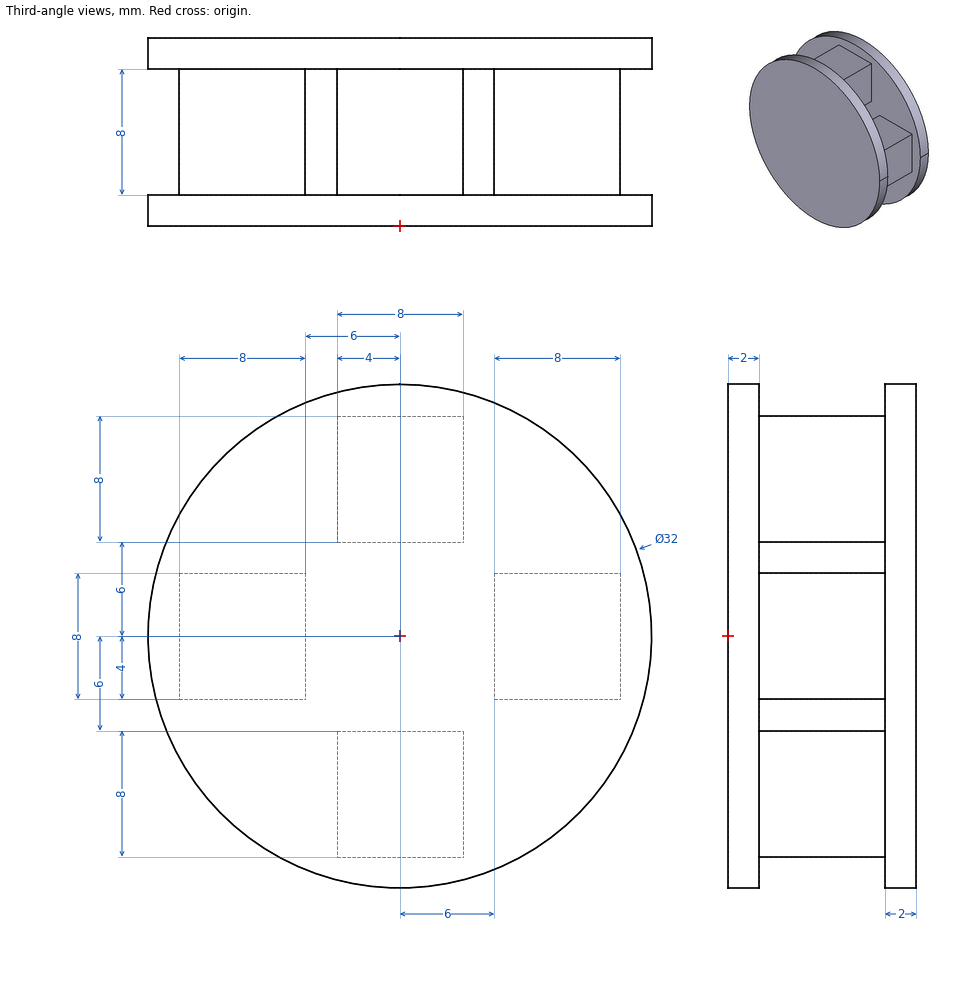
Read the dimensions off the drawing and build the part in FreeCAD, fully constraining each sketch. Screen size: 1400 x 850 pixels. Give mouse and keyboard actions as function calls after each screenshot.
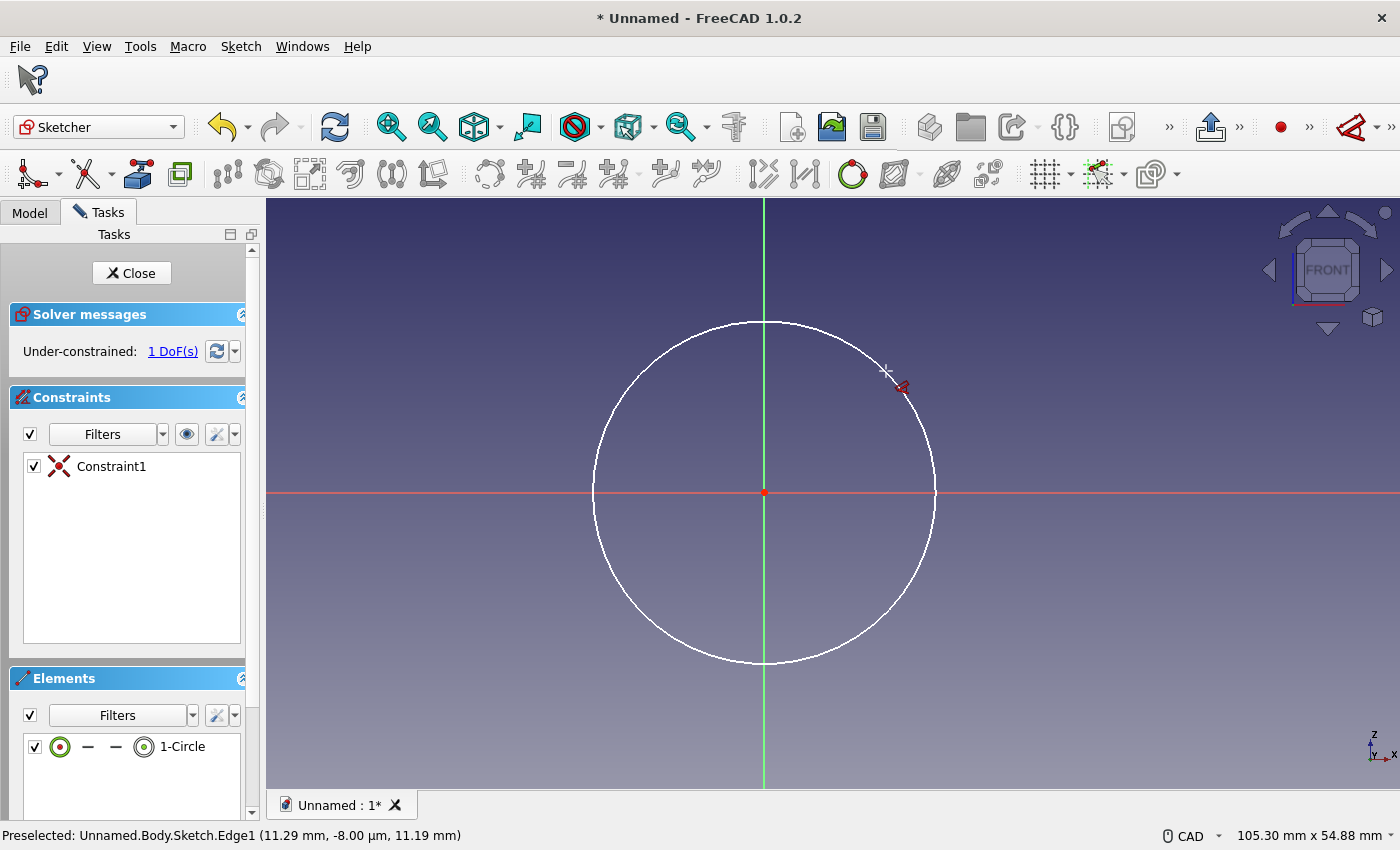
click(885, 371)
click(908, 348)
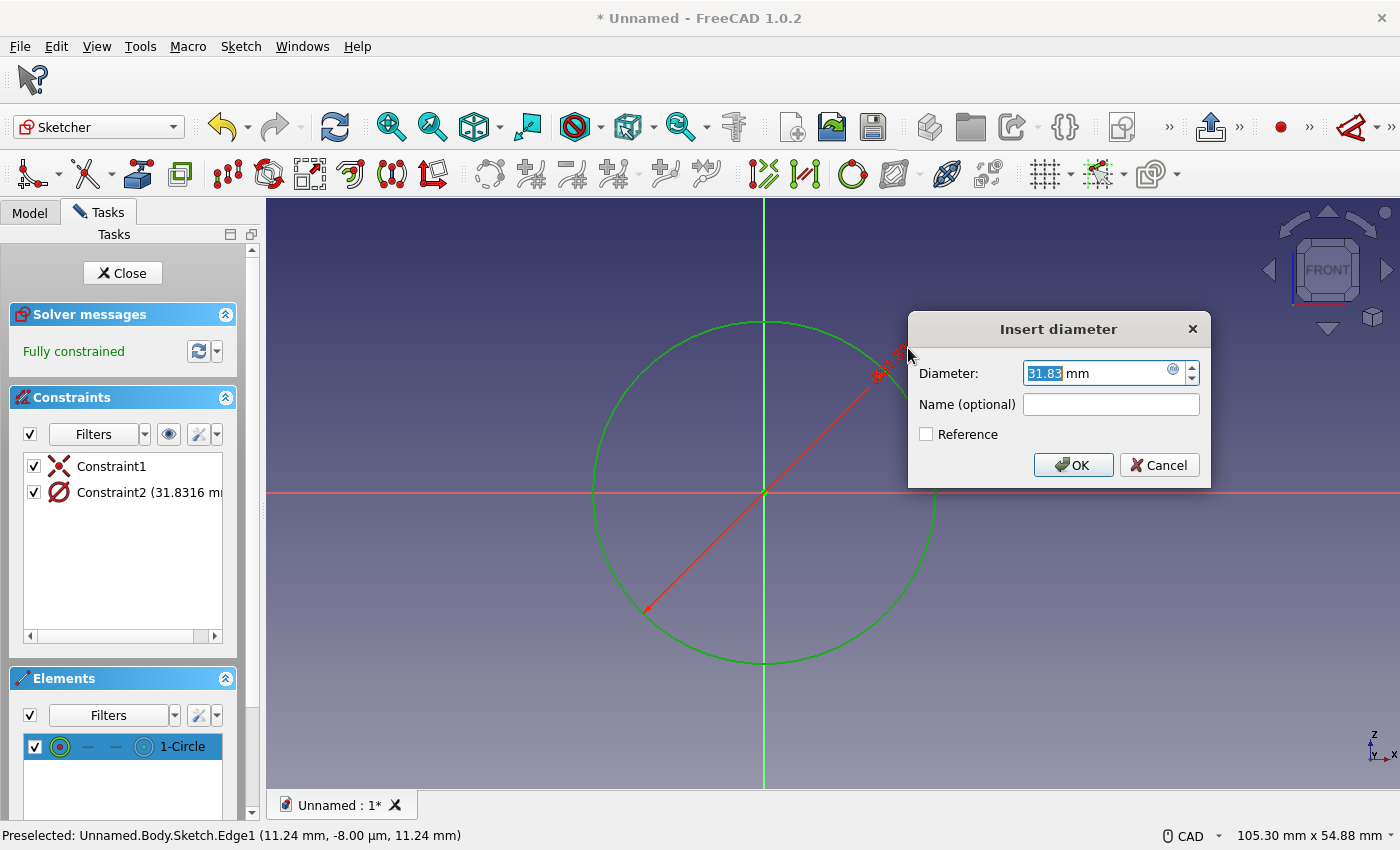
text(32)
key(Return)
key(Escape)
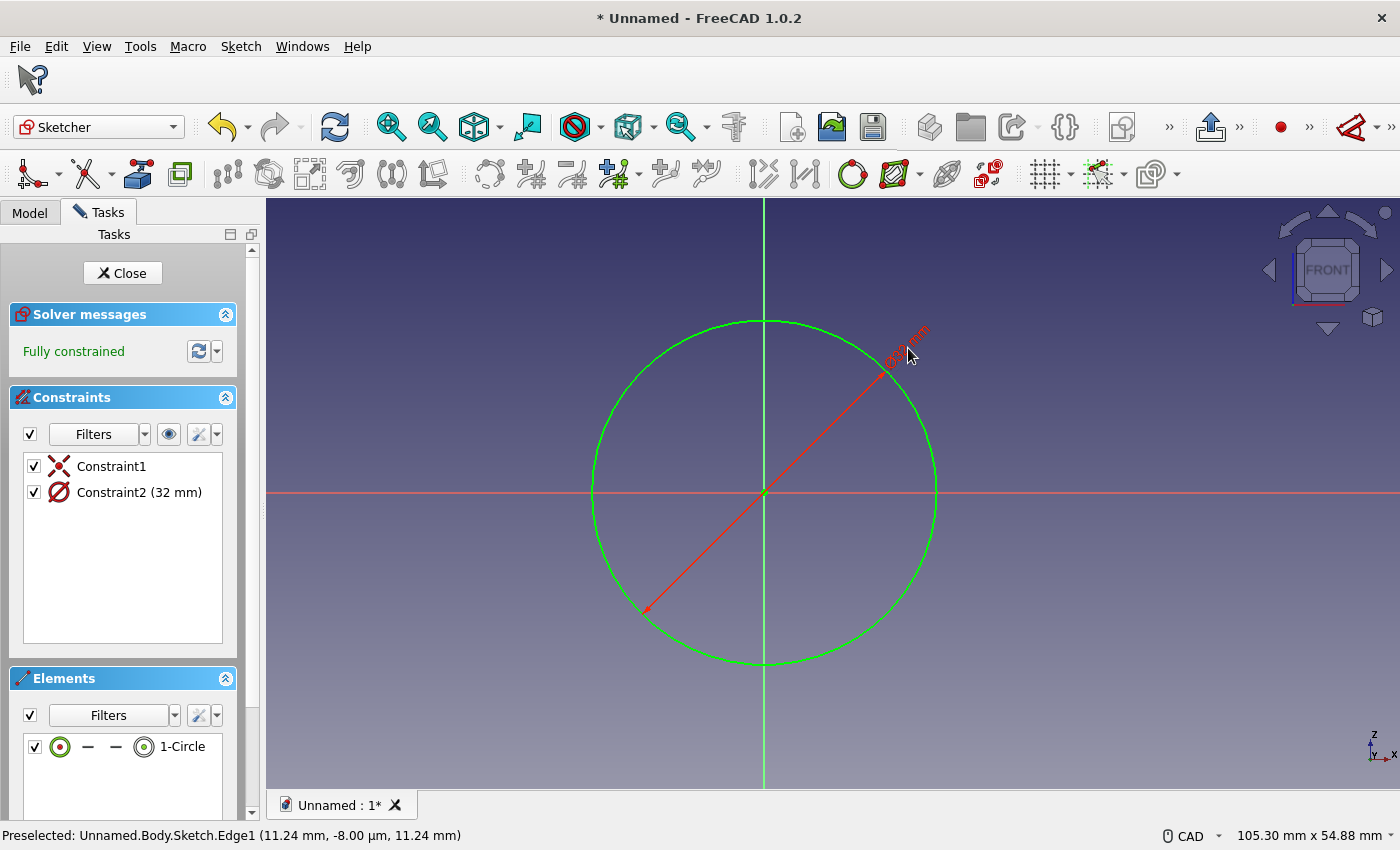
click(123, 273)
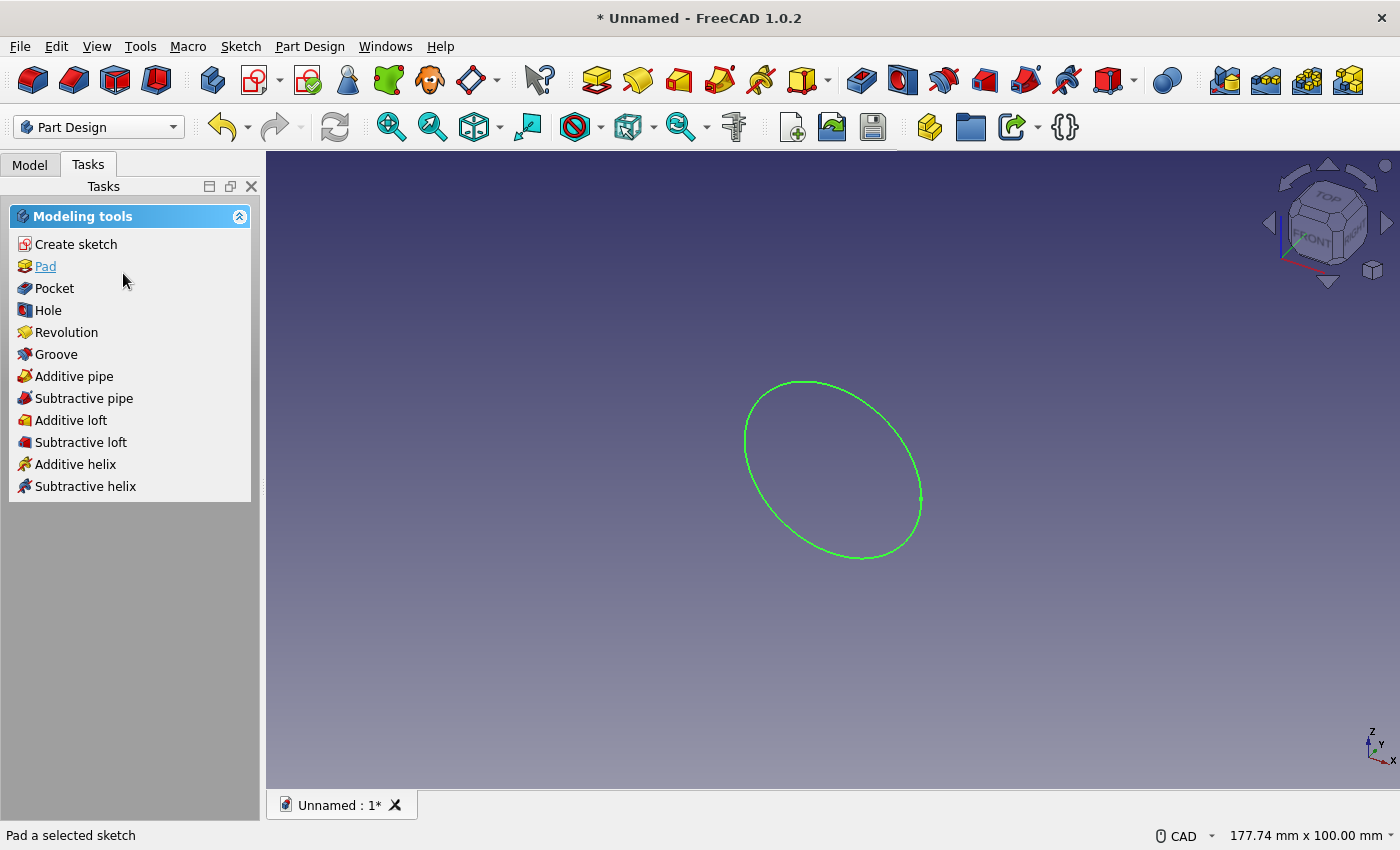
click(597, 80)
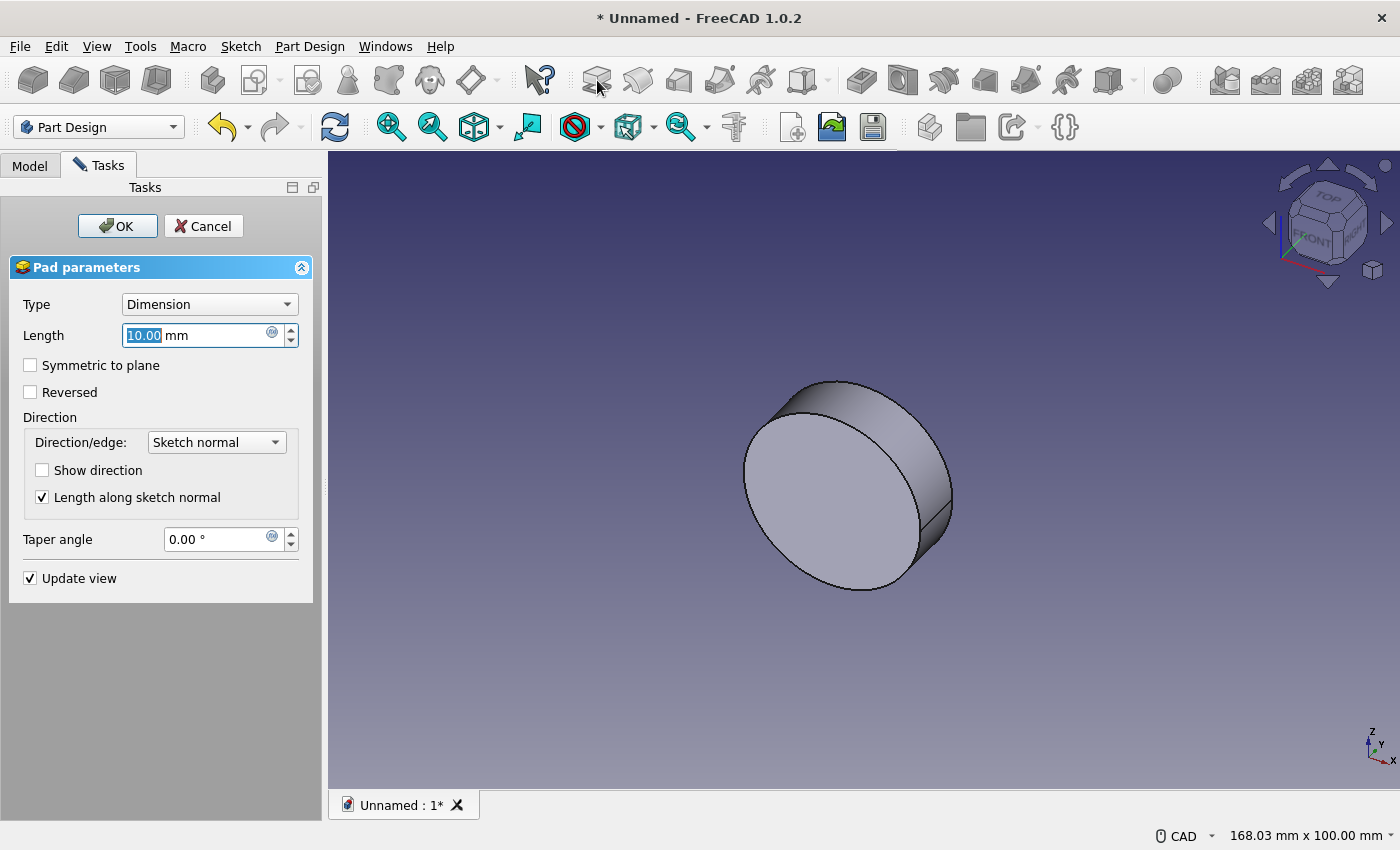
text(2)
key(Tab)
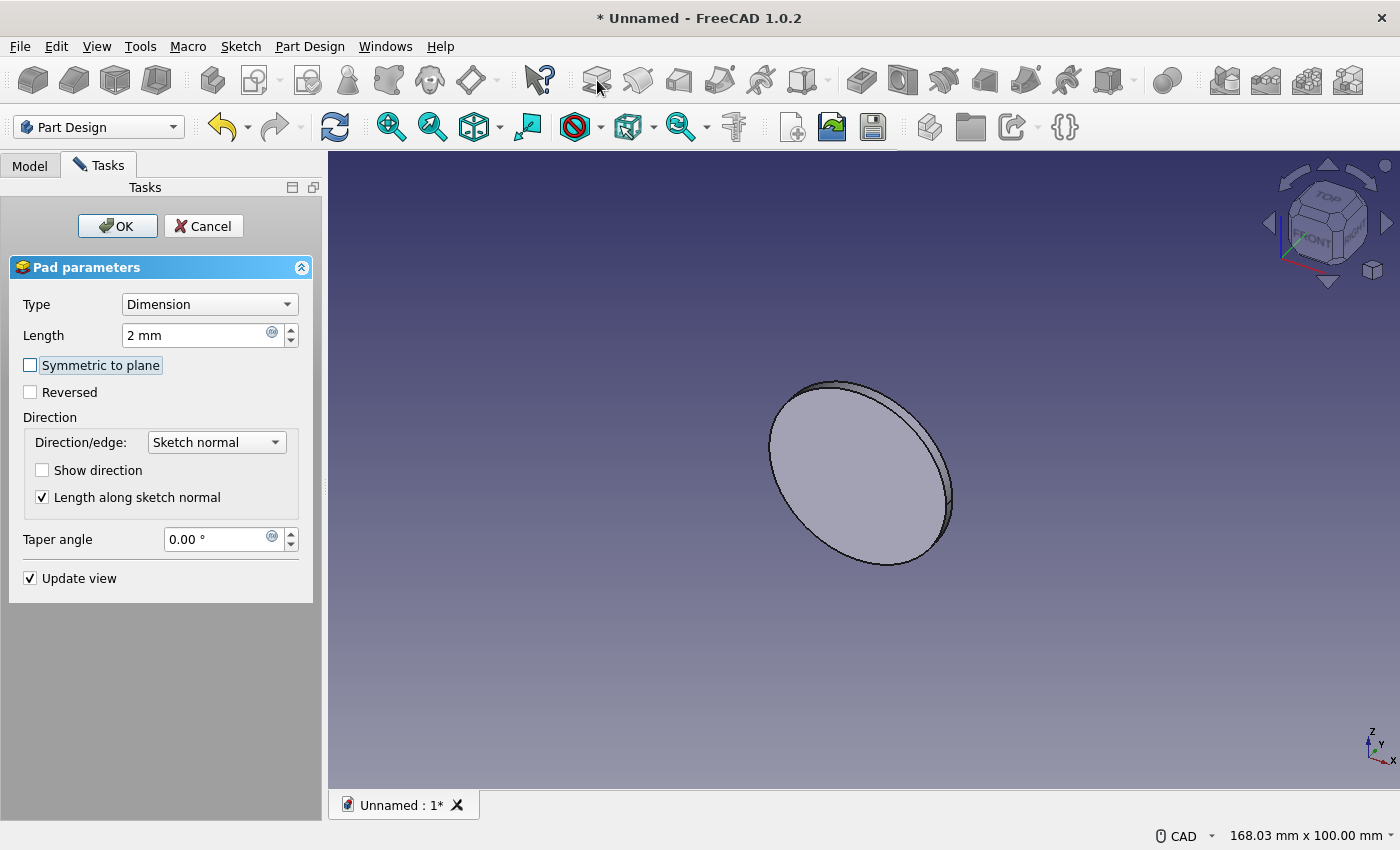
click(31, 392)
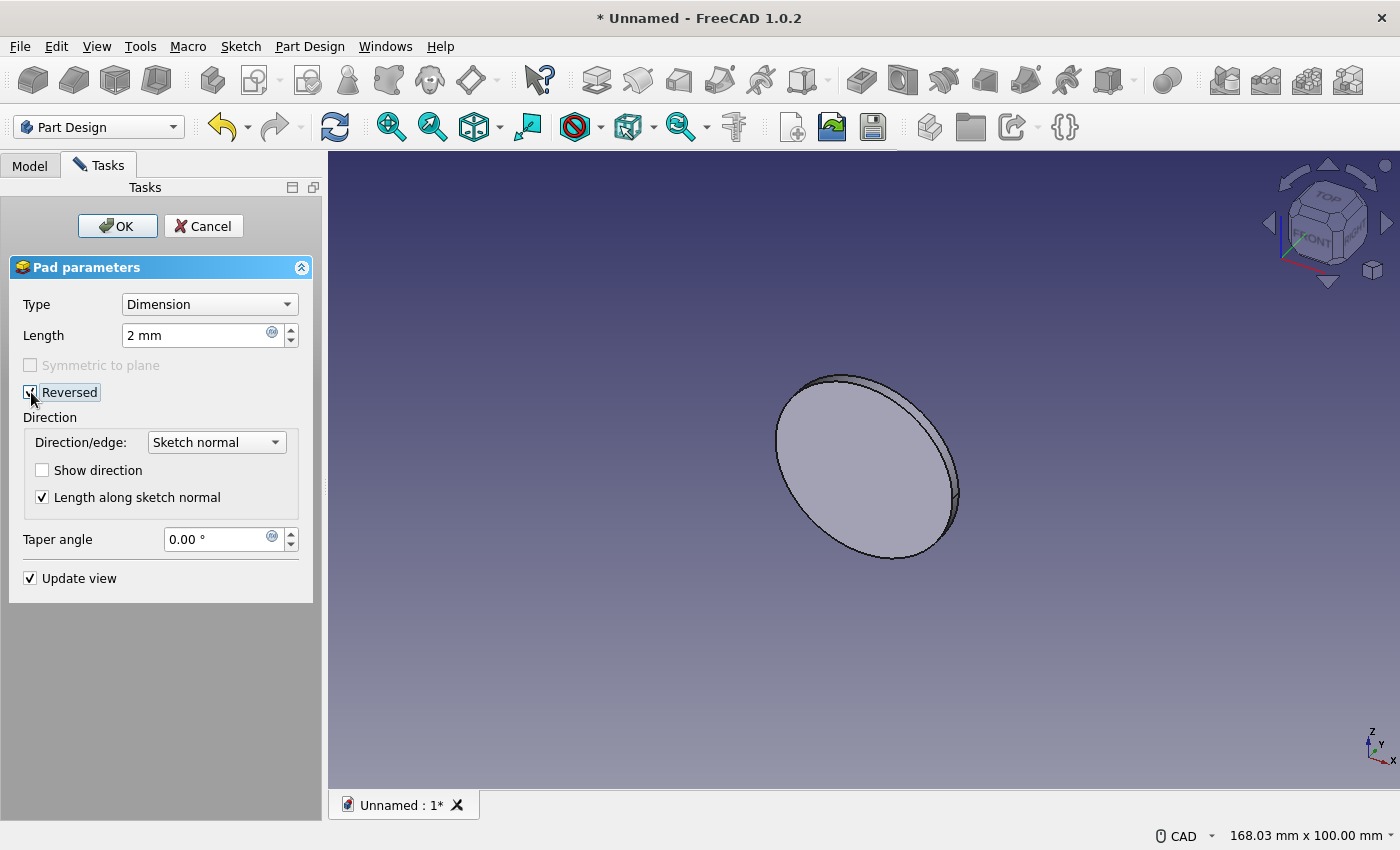
click(118, 226)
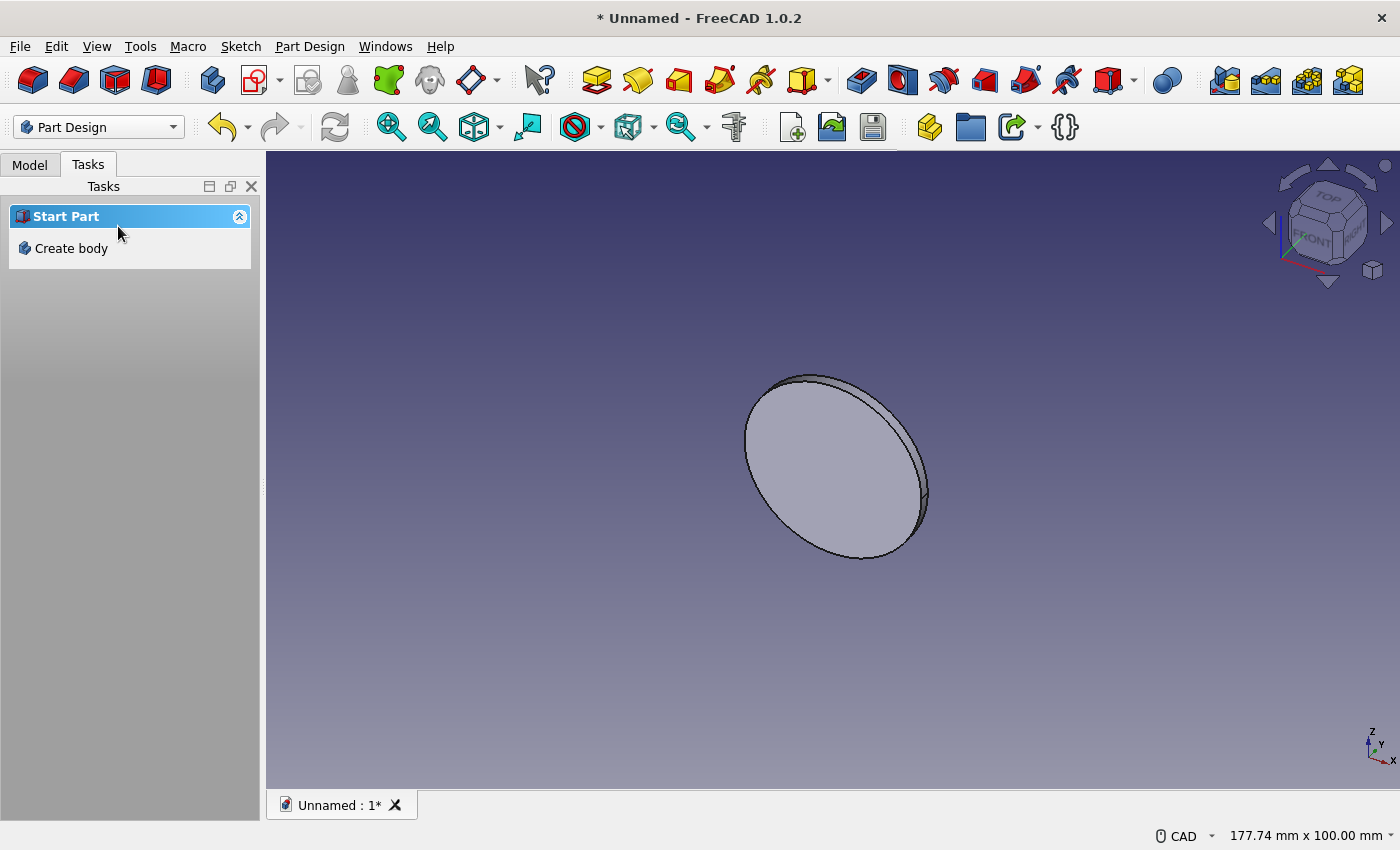
key(v)
key(f)